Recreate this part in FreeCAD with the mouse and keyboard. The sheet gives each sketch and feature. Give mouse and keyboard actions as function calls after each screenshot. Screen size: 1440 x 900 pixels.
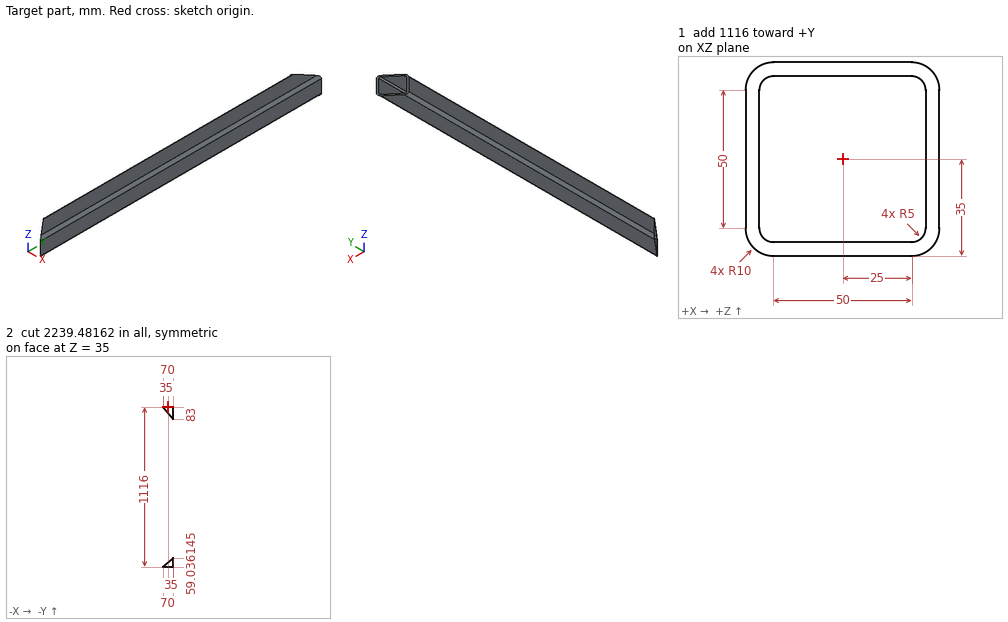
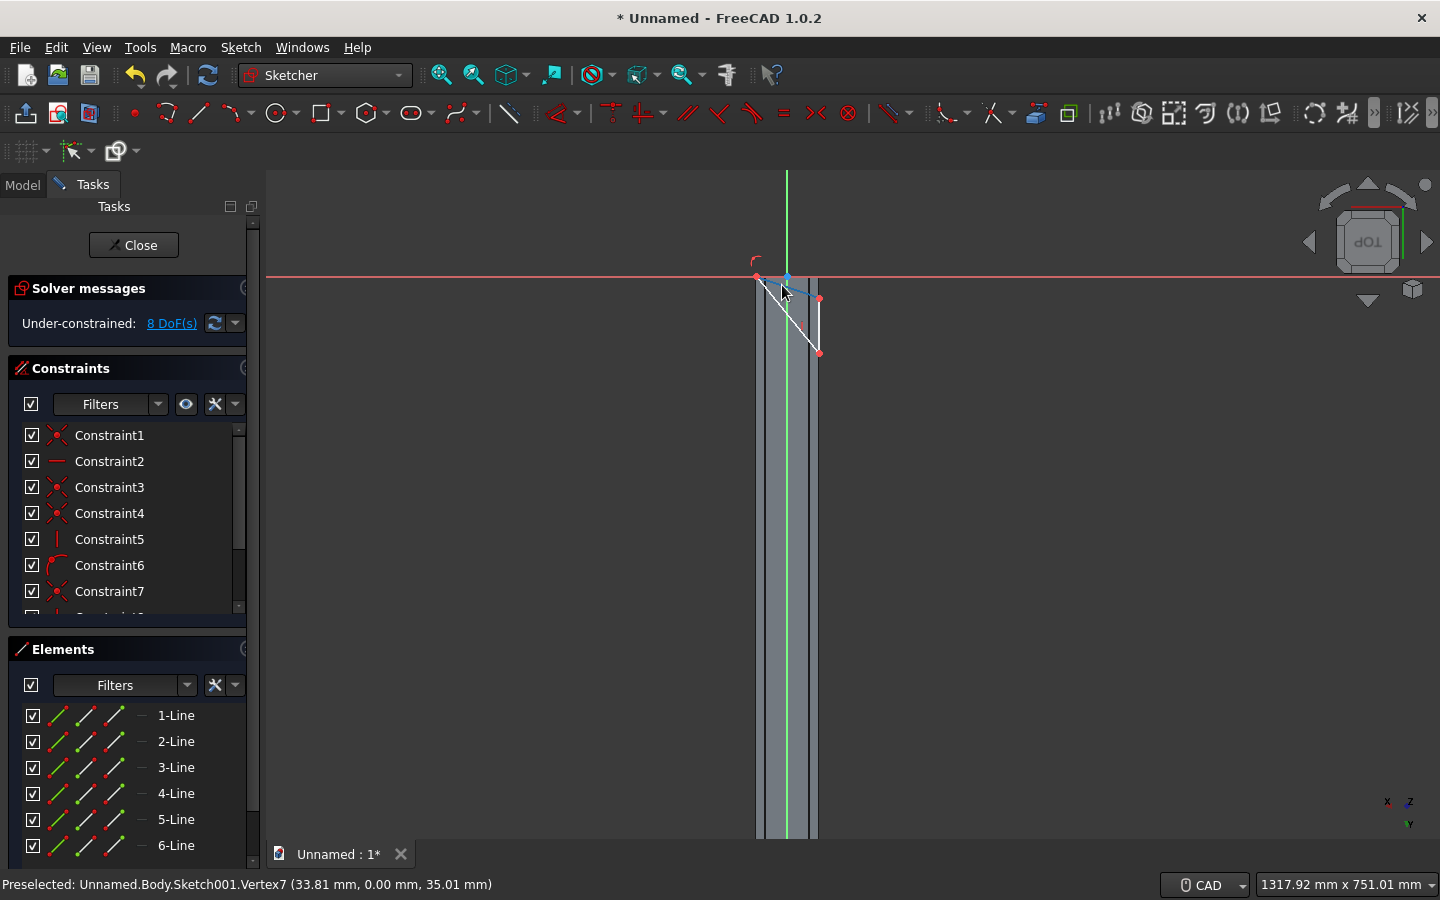
click(782, 285)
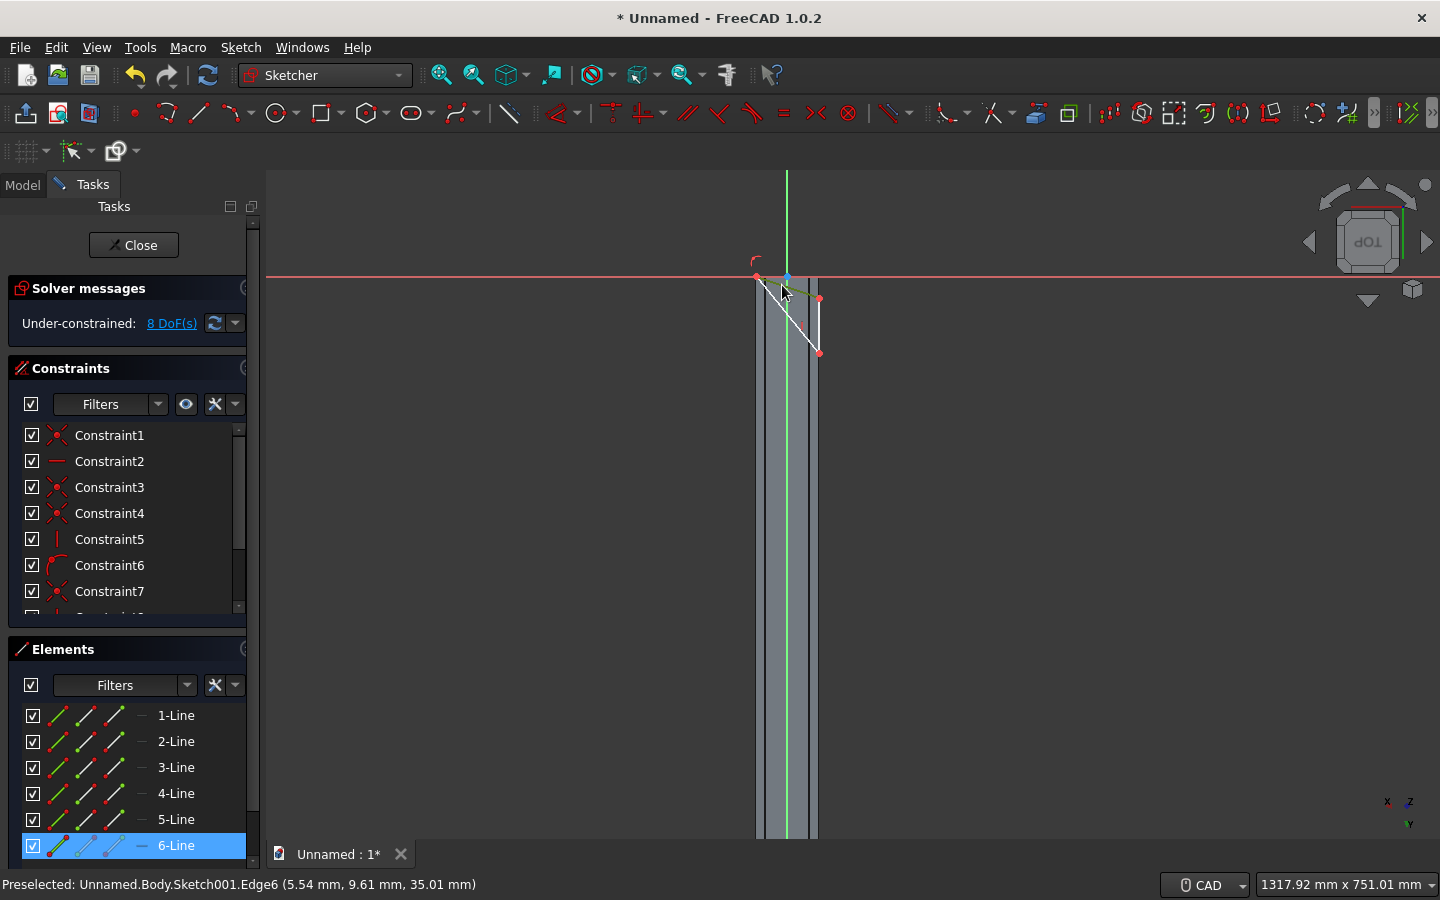
key(h)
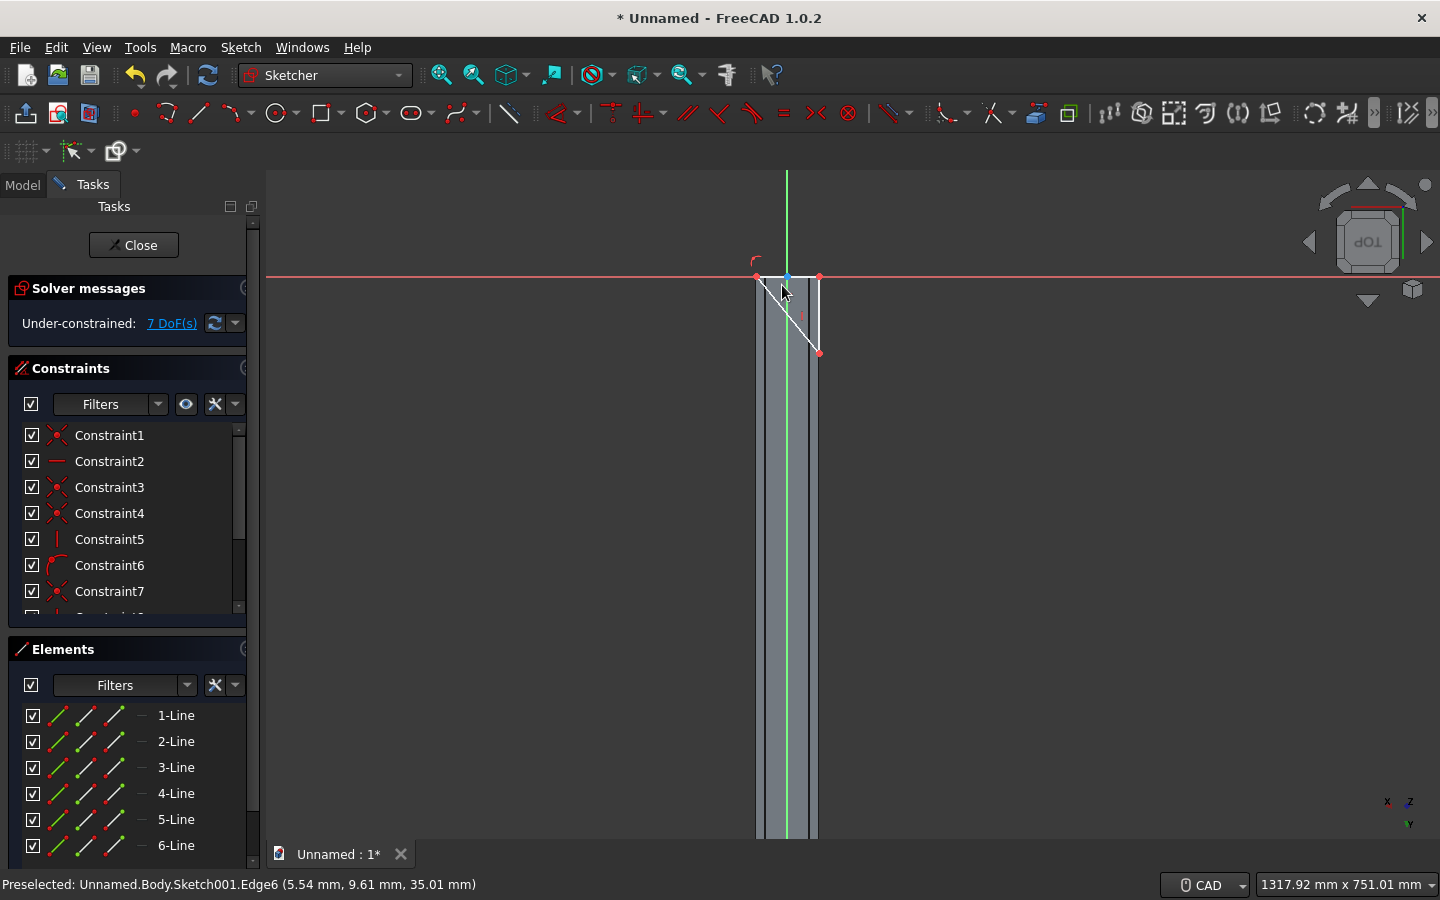
key(d)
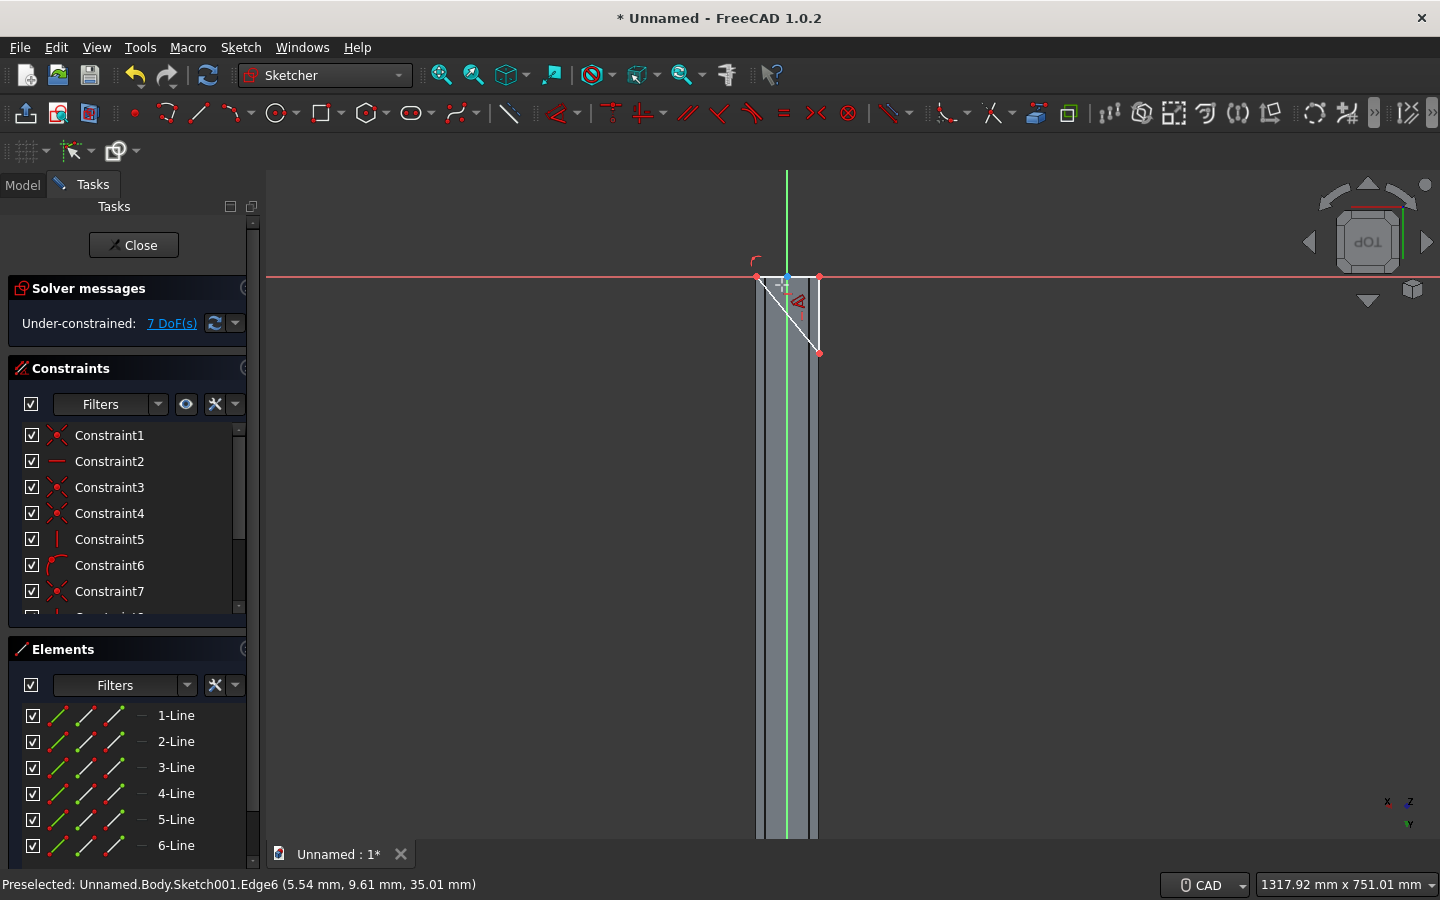
scroll(782, 285, down, 4)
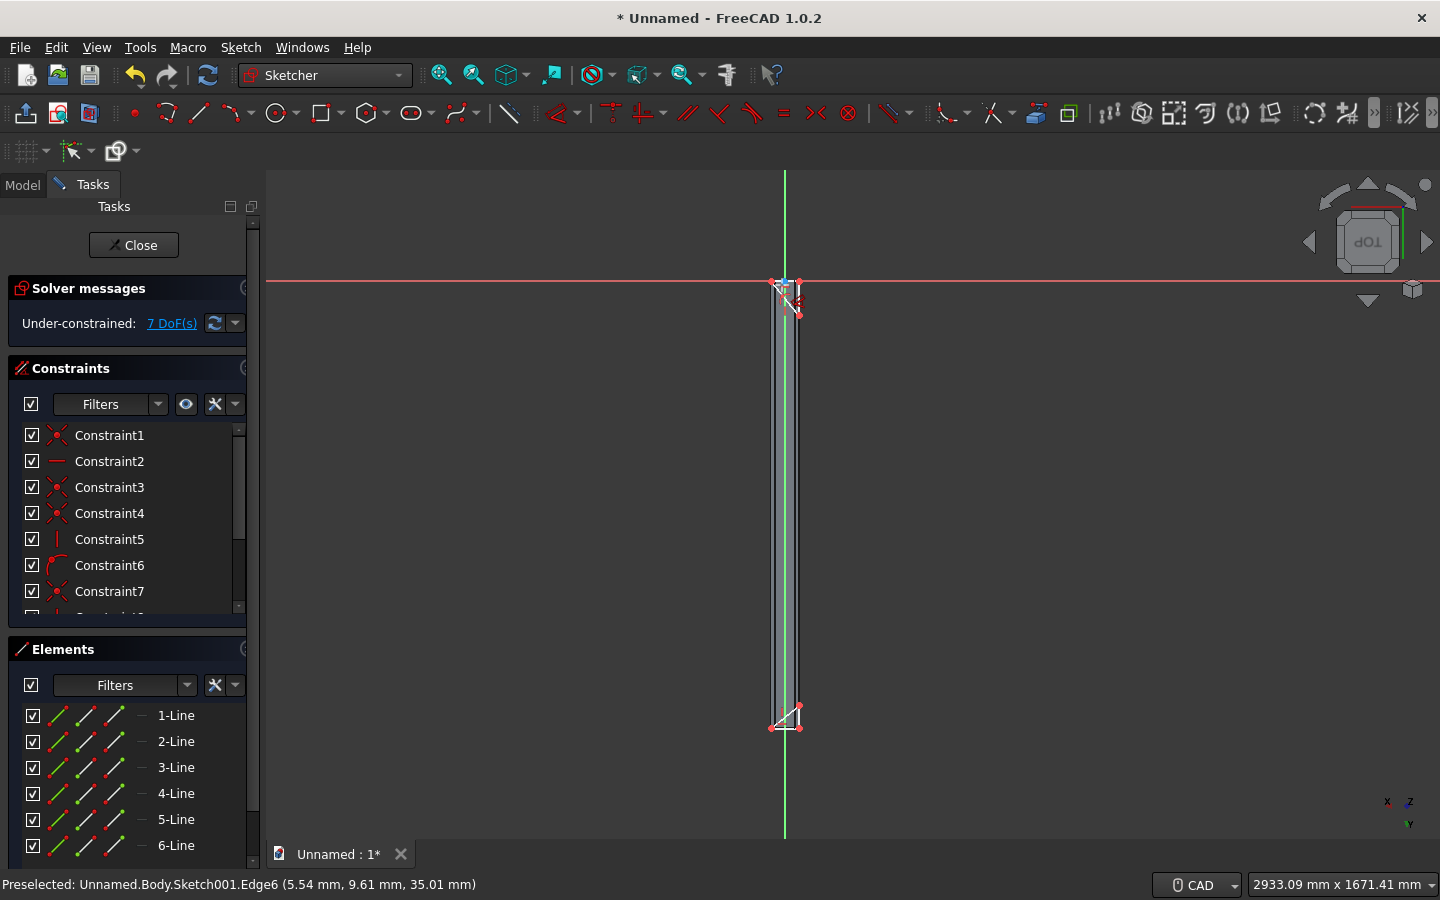
scroll(779, 729, up, 5)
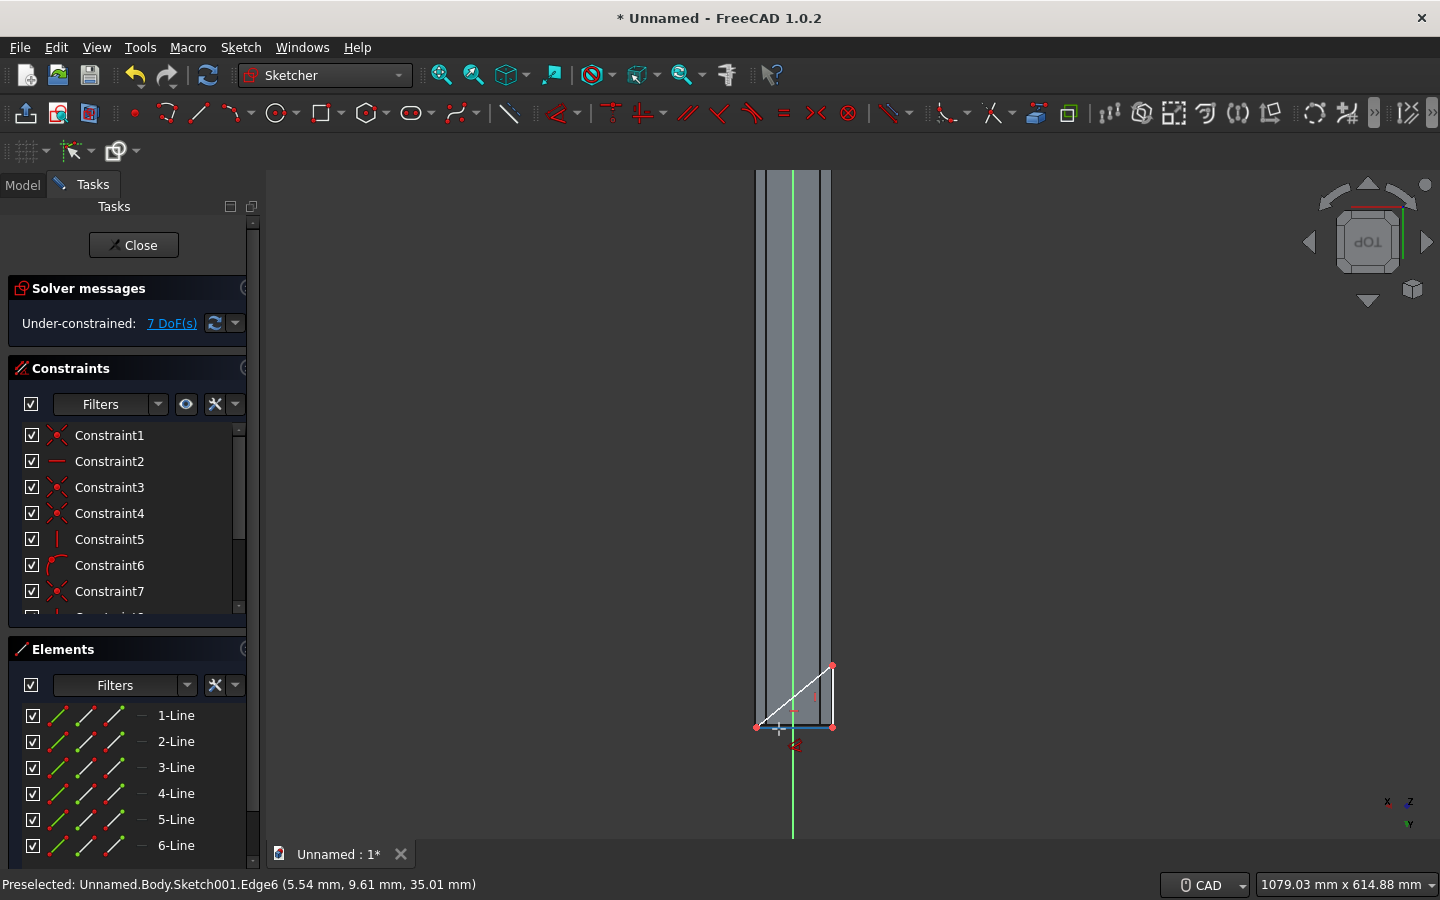
click(779, 728)
click(777, 762)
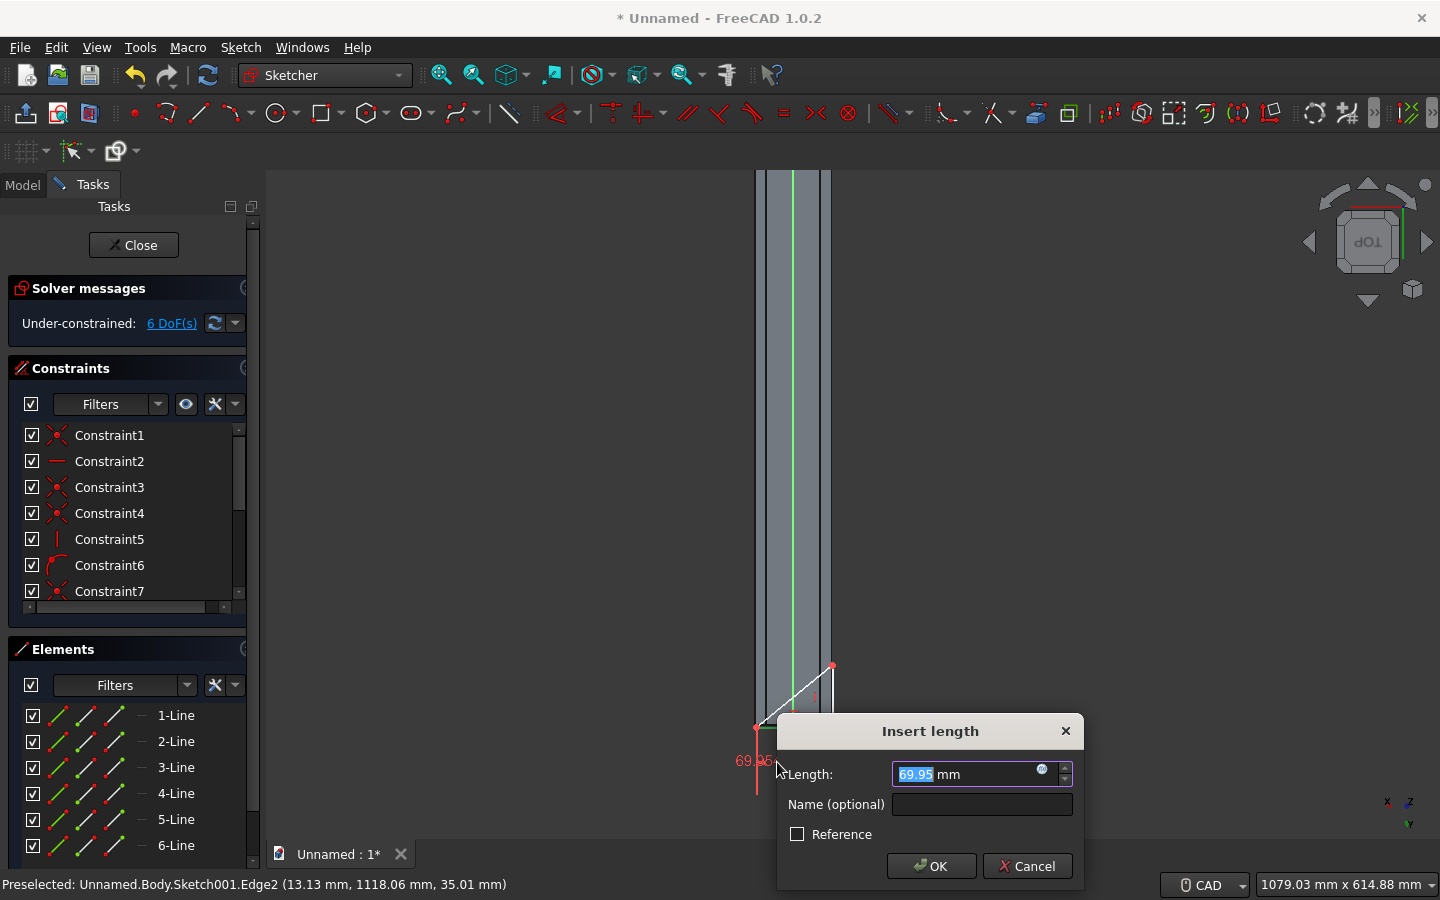
text(70)
key(Return)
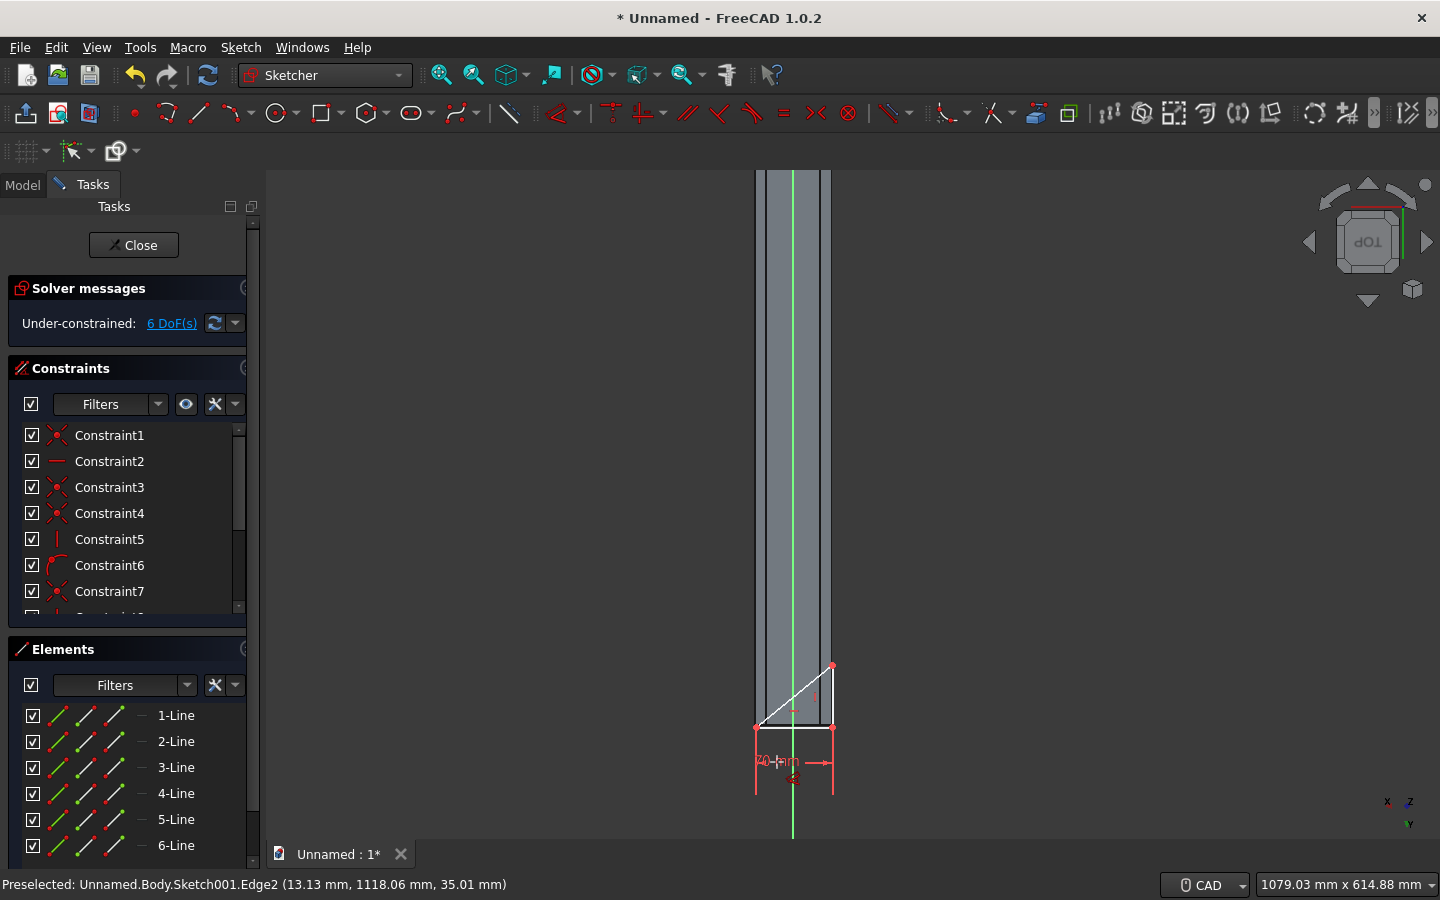
scroll(779, 729, down, 5)